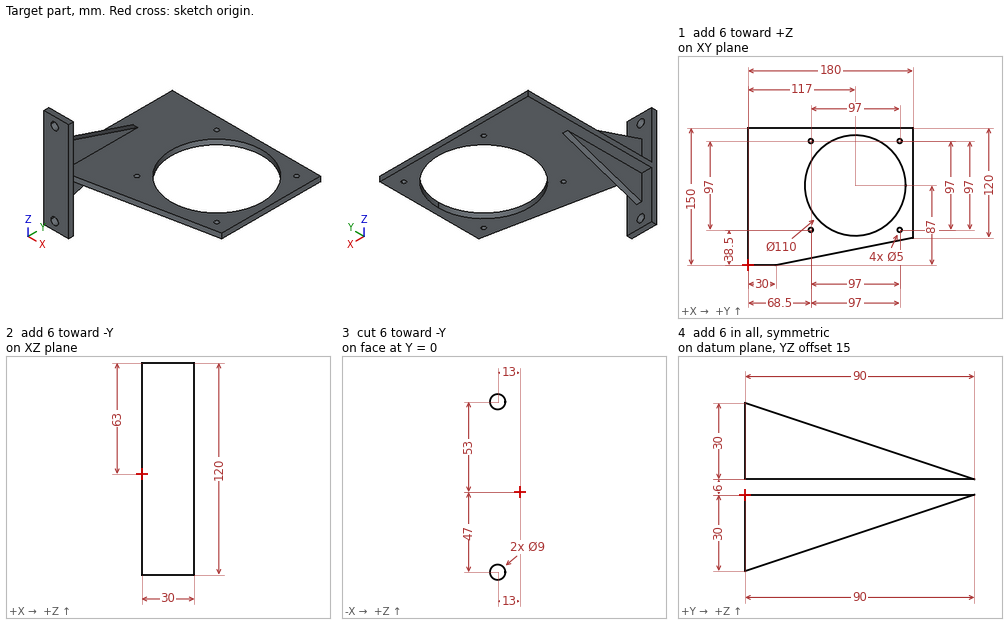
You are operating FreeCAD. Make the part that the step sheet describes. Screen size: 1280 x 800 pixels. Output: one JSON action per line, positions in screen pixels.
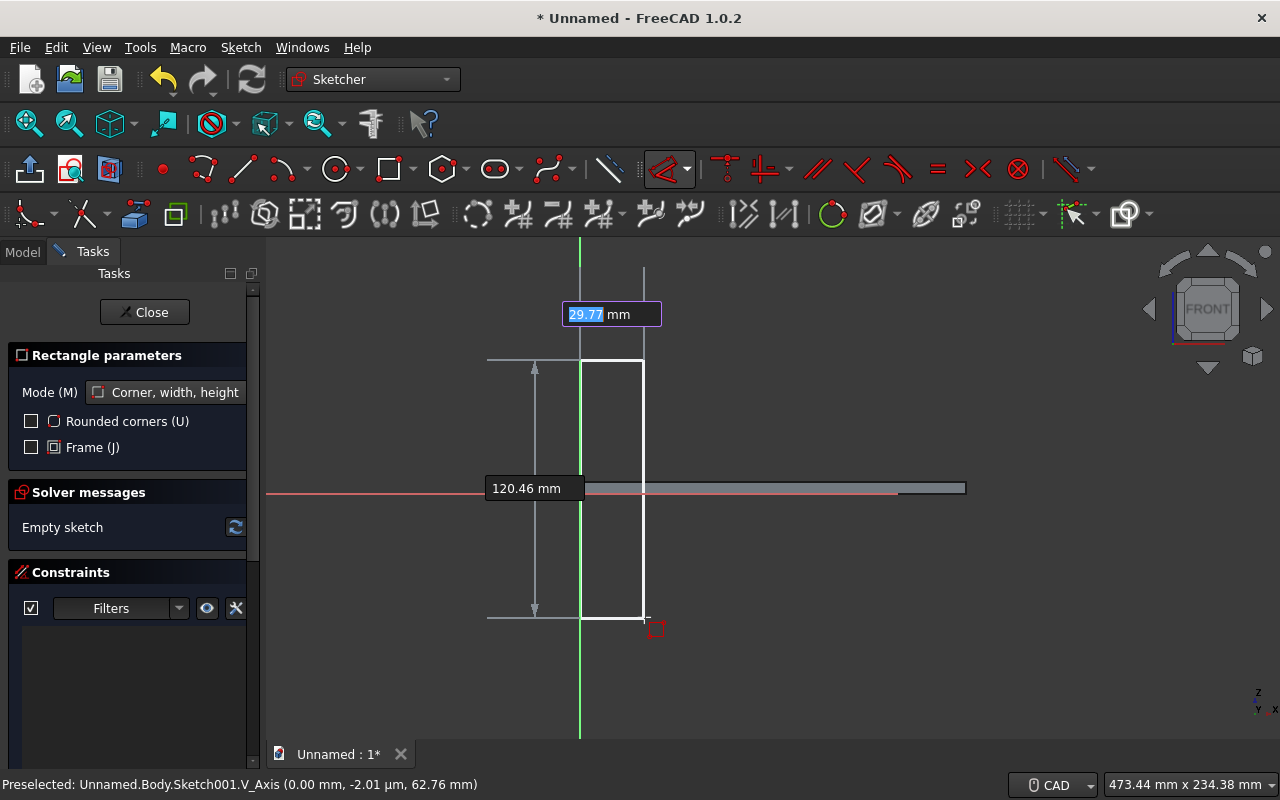
{"action": "type", "text": "30"}
{"action": "key", "text": "Tab"}
{"action": "type", "text": "120"}
{"action": "key", "text": "Return"}
{"action": "key", "text": "Escape"}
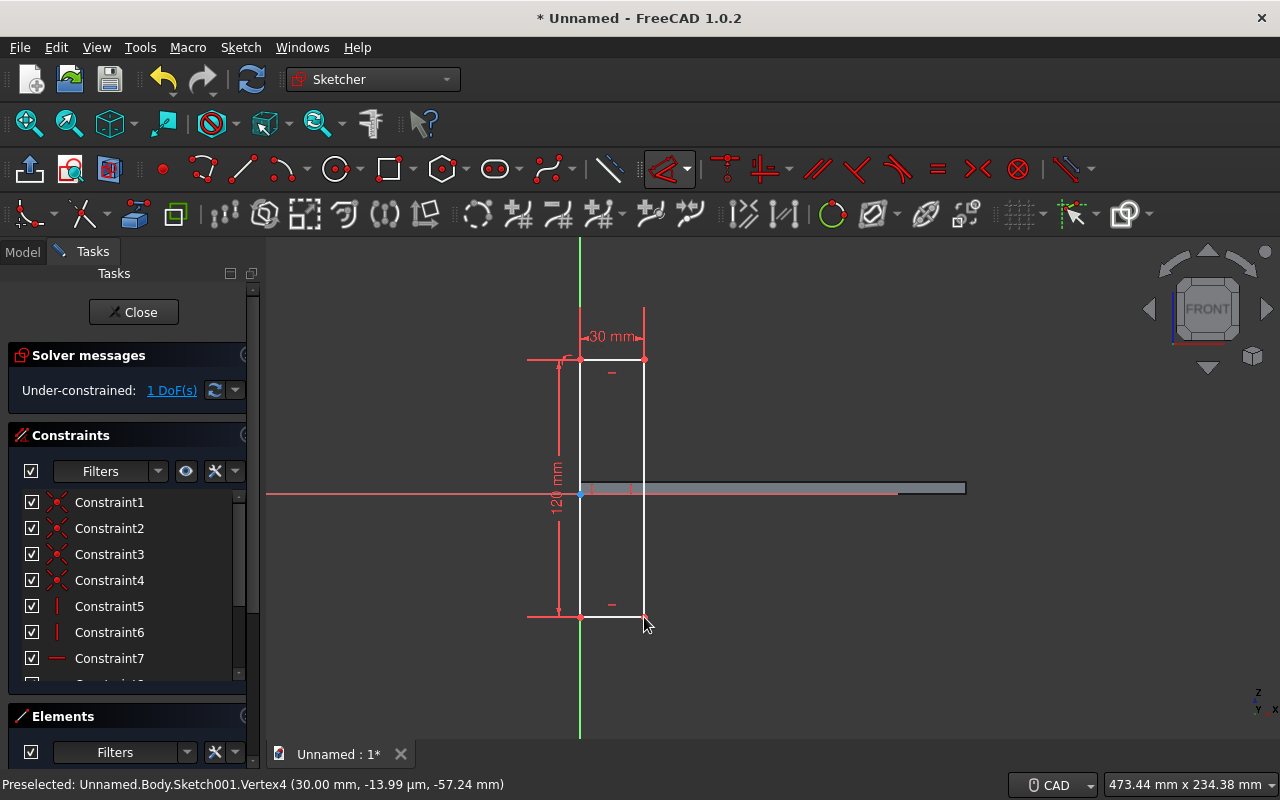
{"action": "left_click", "coordinate": [580, 360]}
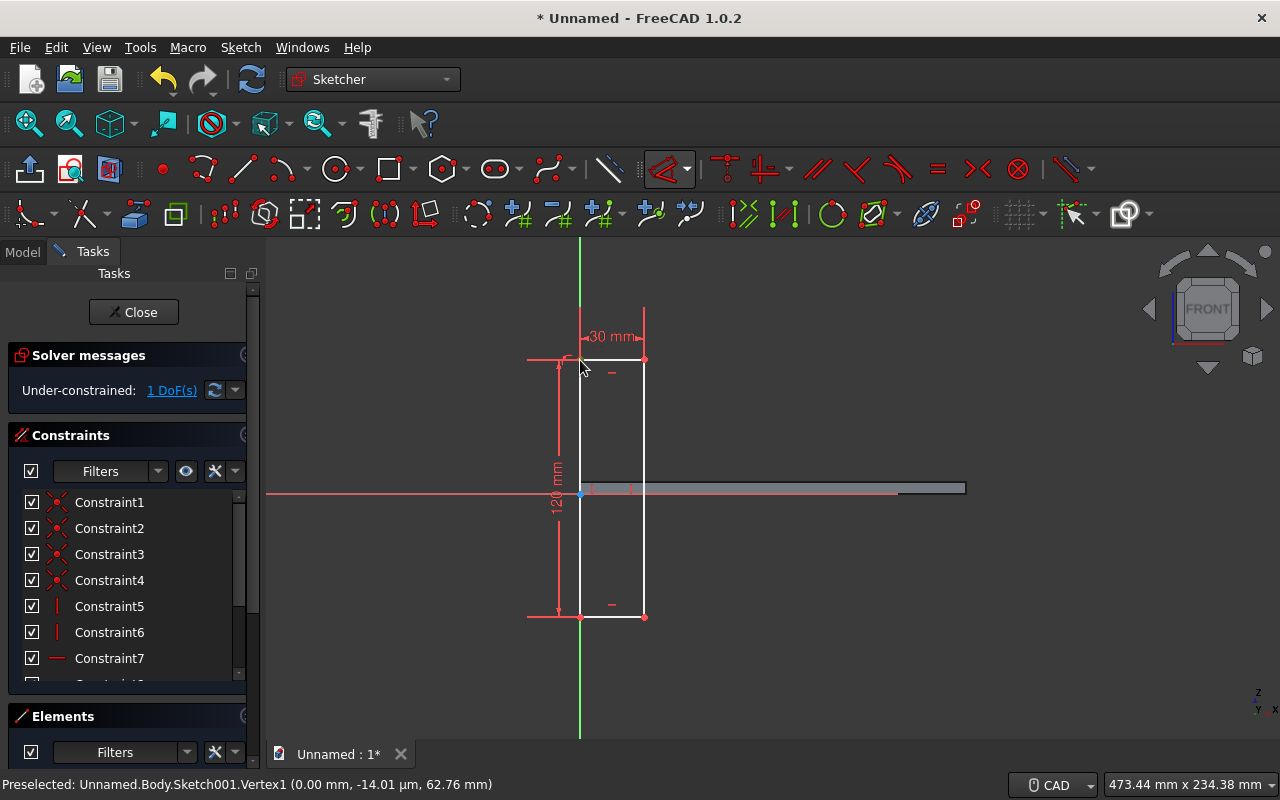
{"action": "key", "text": "i"}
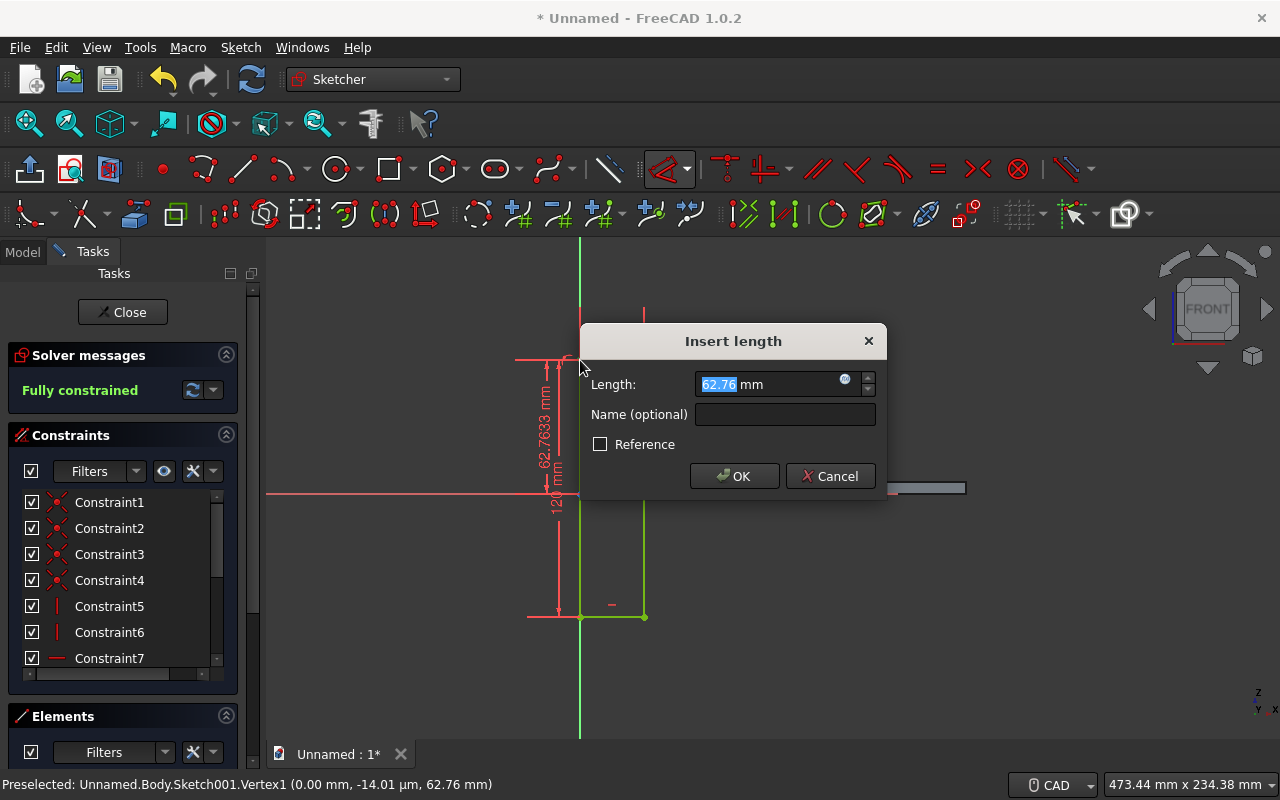
{"action": "type", "text": "63"}
{"action": "key", "text": "Return"}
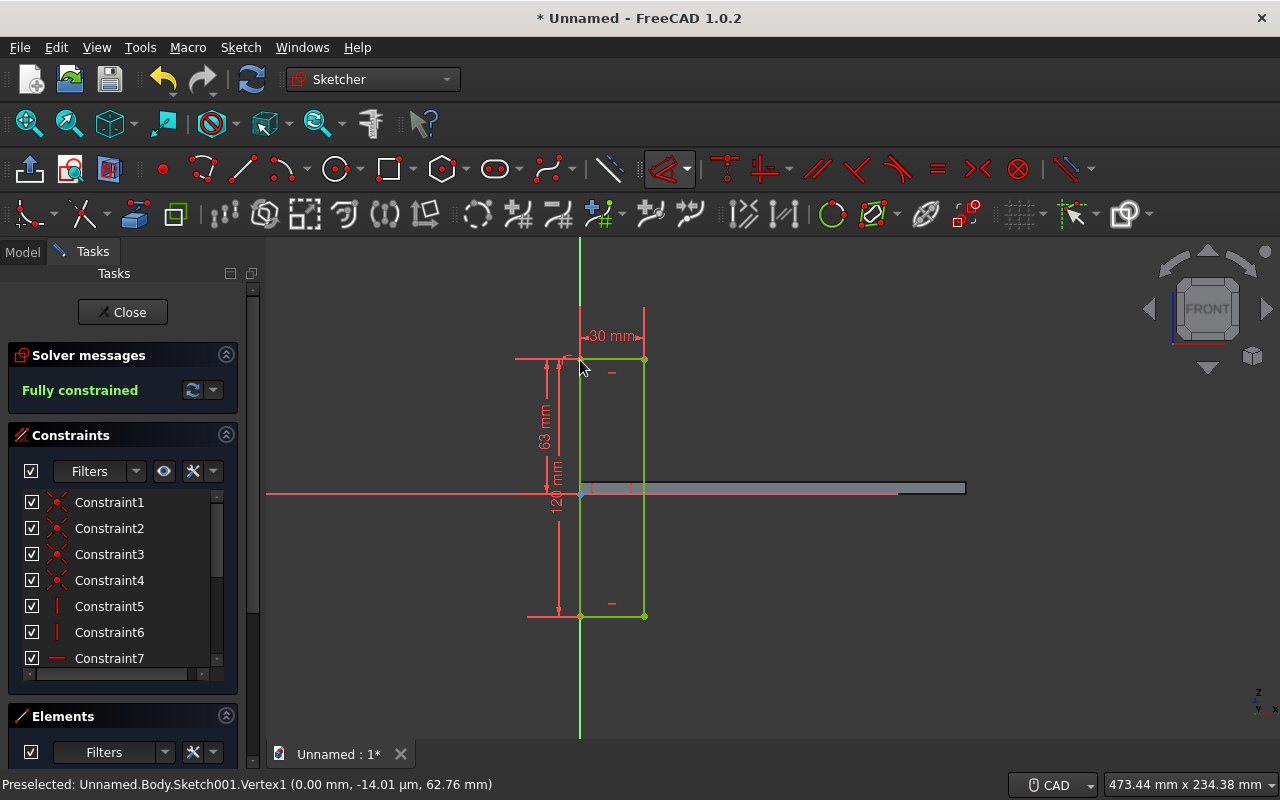
{"action": "left_click", "coordinate": [123, 312]}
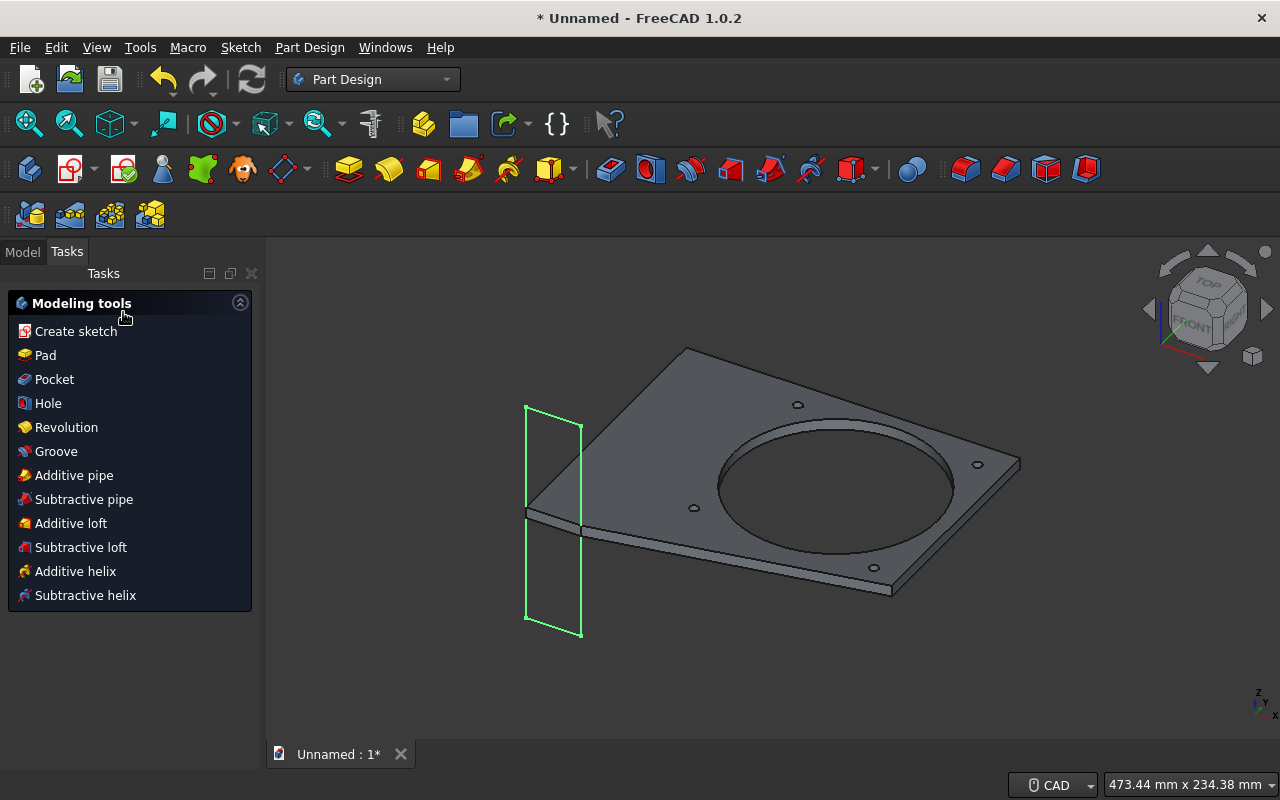
{"action": "left_click", "coordinate": [350, 170]}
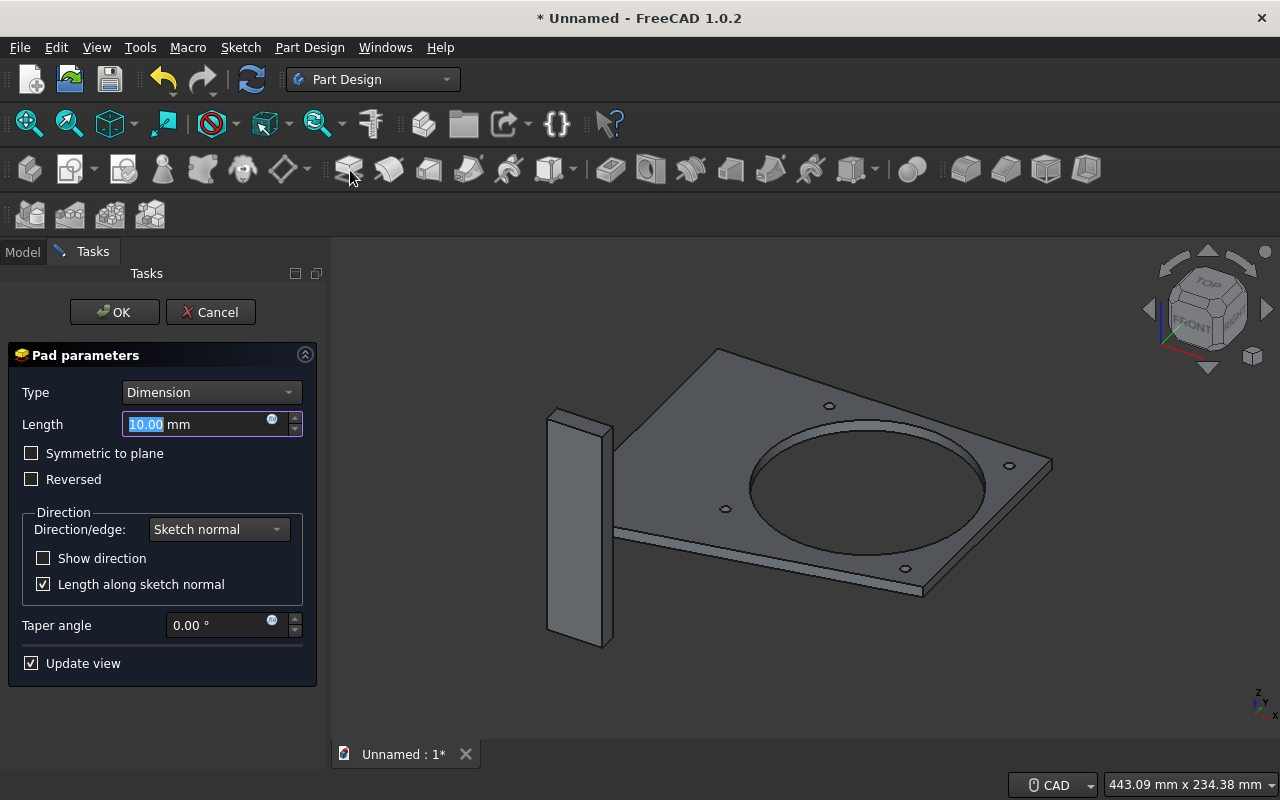
{"action": "type", "text": "6"}
{"action": "key", "text": "Tab"}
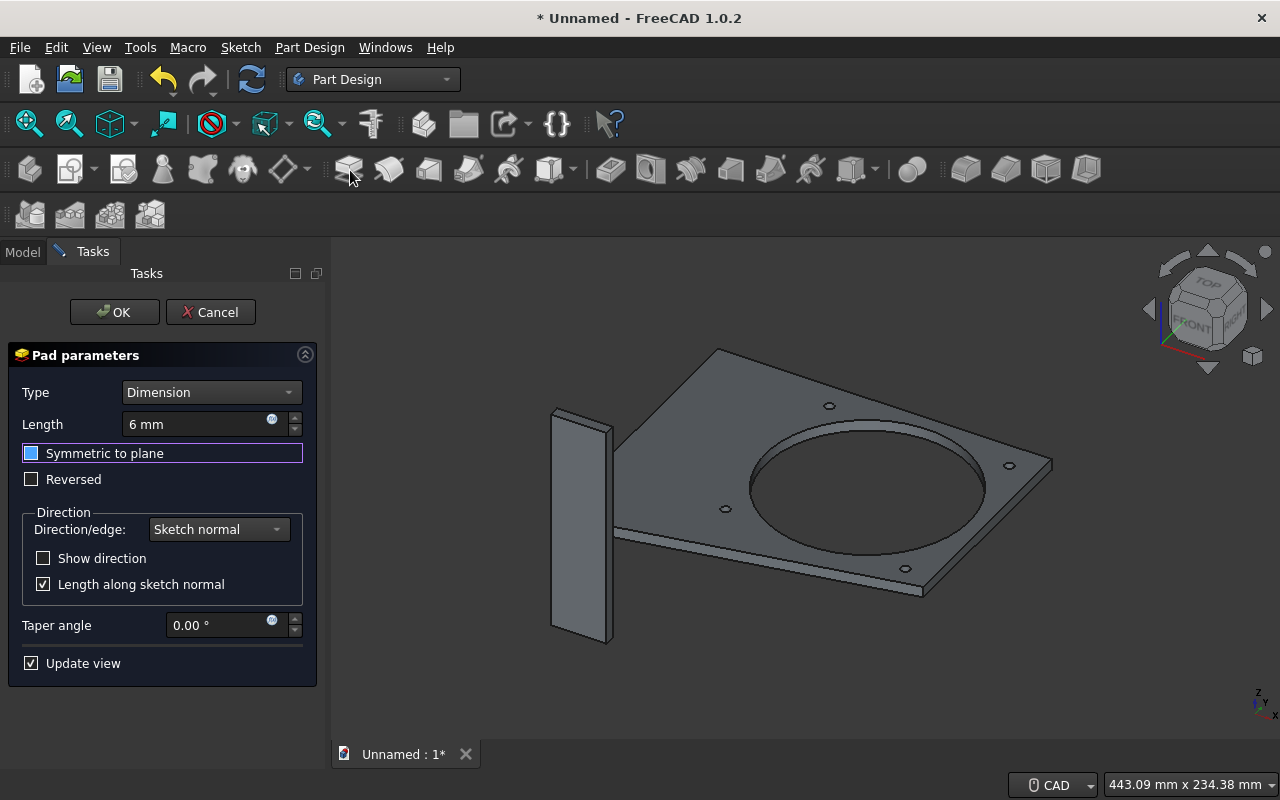
{"action": "left_click", "coordinate": [115, 312]}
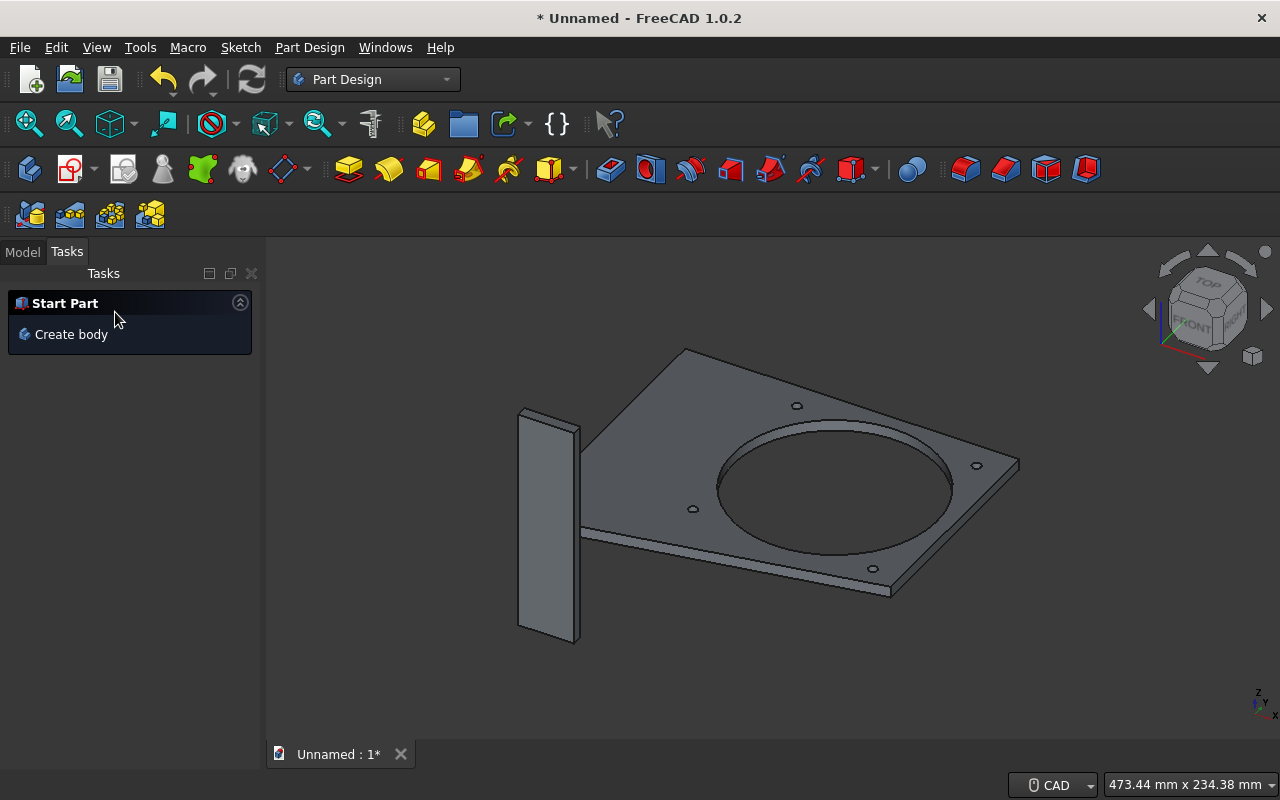
{"action": "key", "text": "4"}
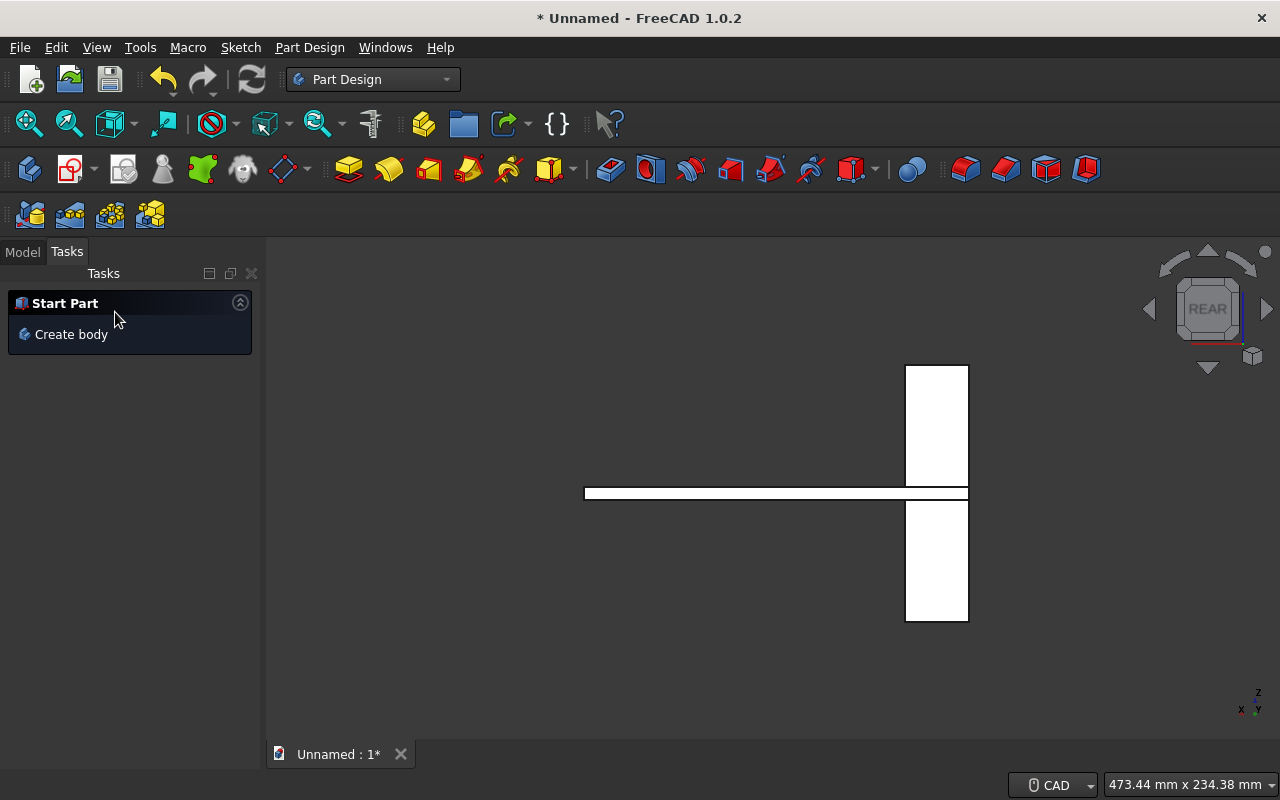
{"action": "left_click", "coordinate": [937, 407]}